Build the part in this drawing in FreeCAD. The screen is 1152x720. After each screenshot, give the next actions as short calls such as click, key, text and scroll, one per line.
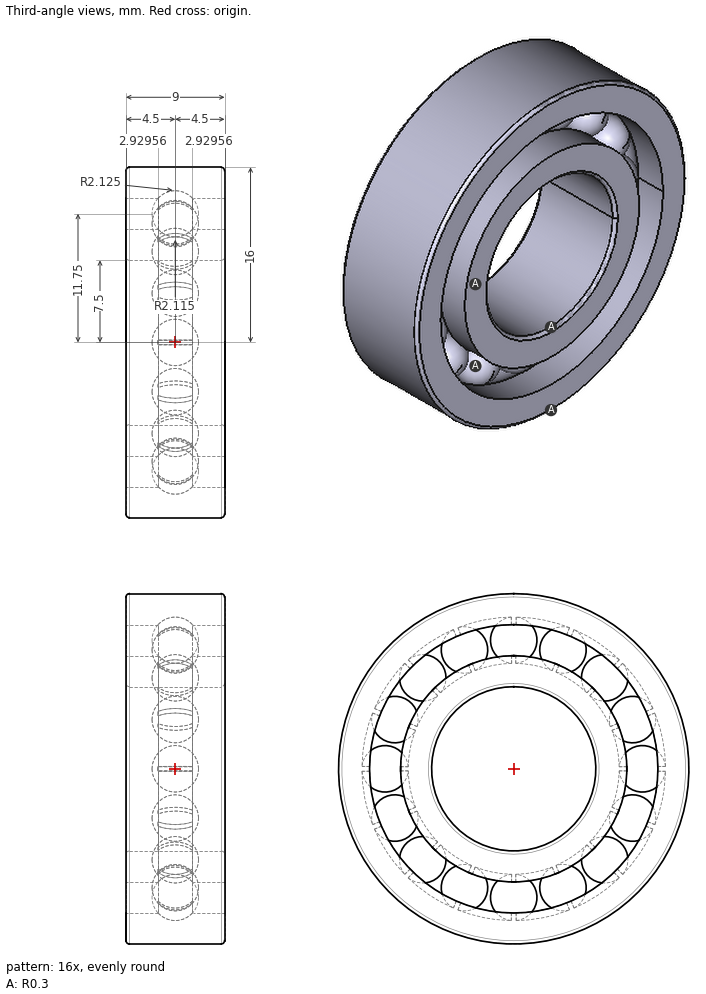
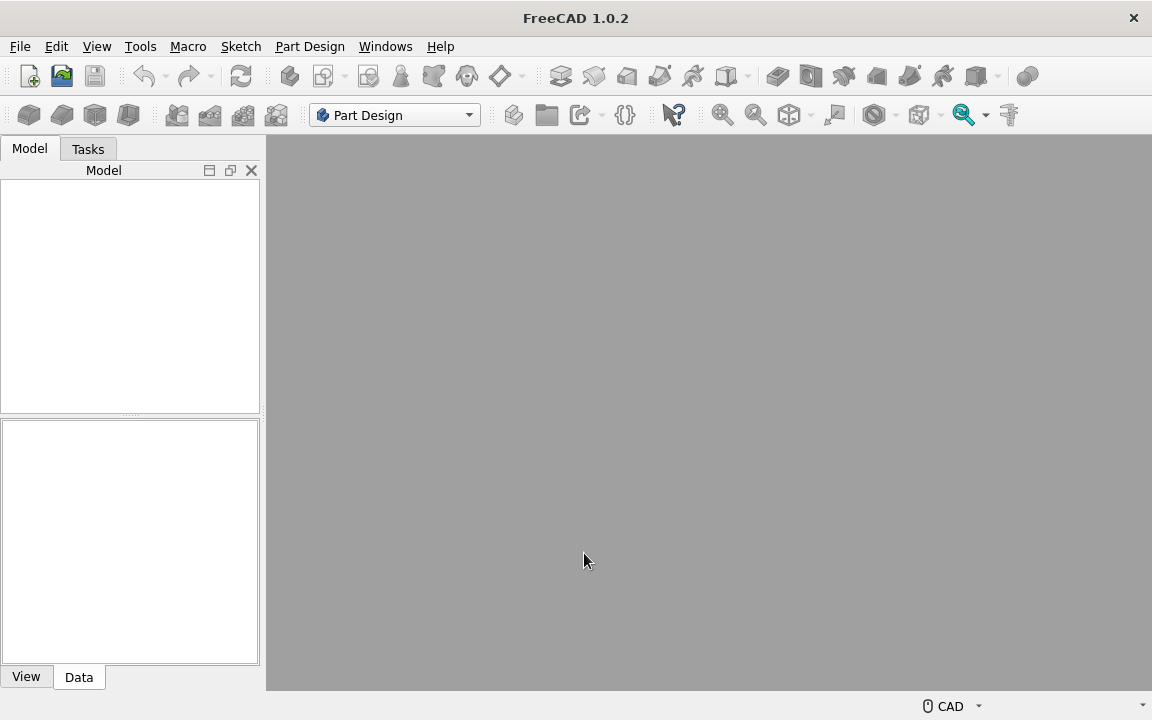
click(29, 76)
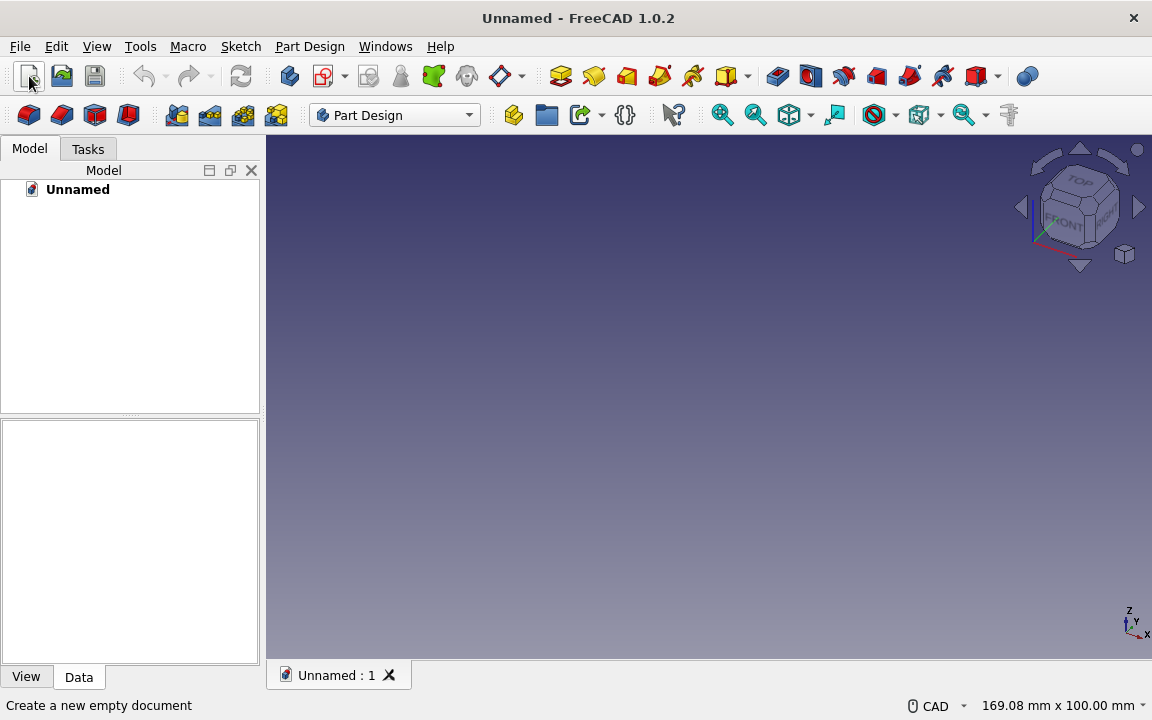
click(322, 76)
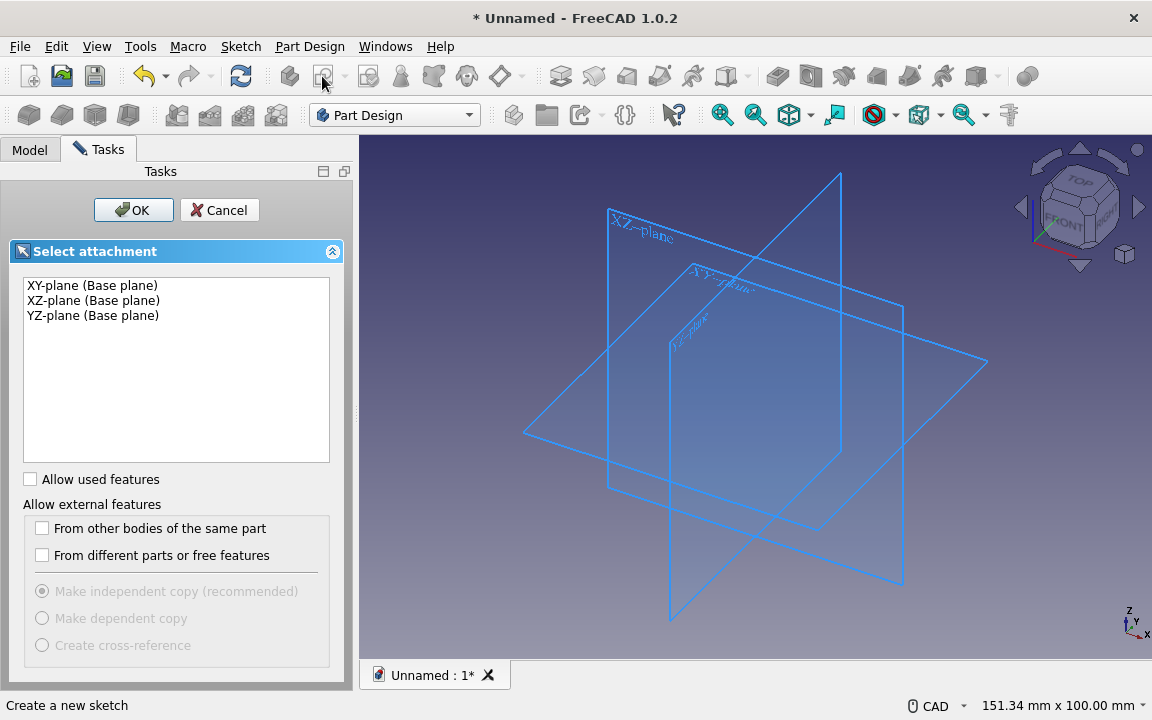
click(84, 286)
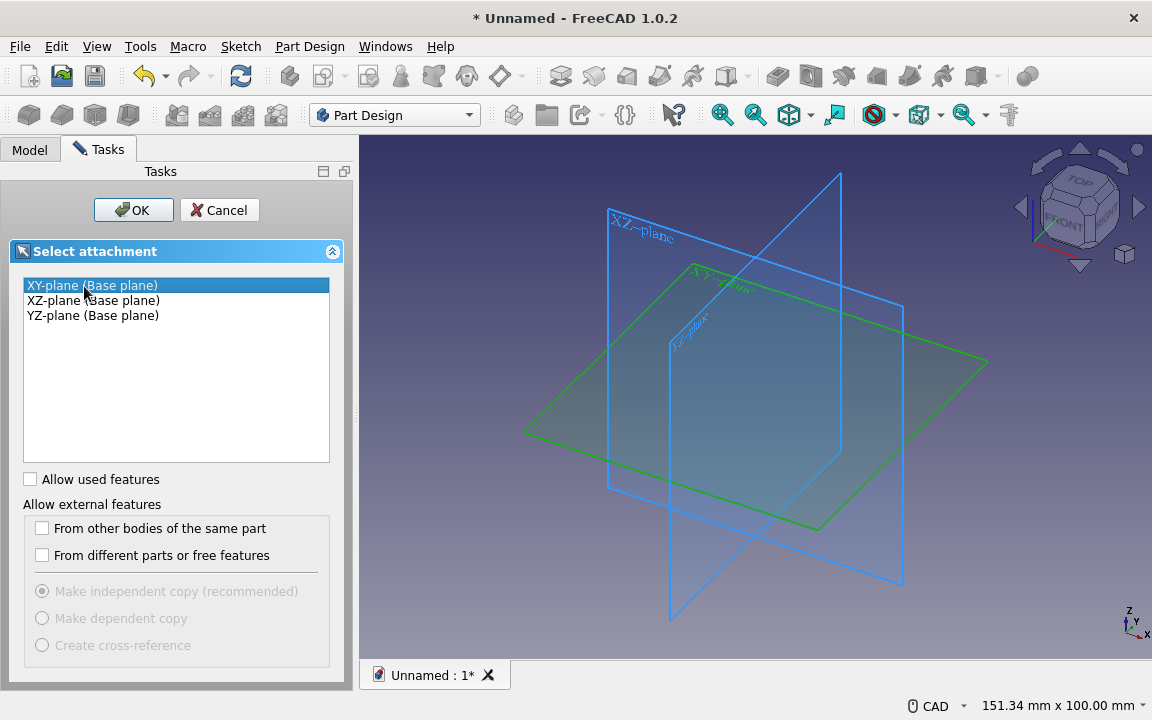
click(134, 210)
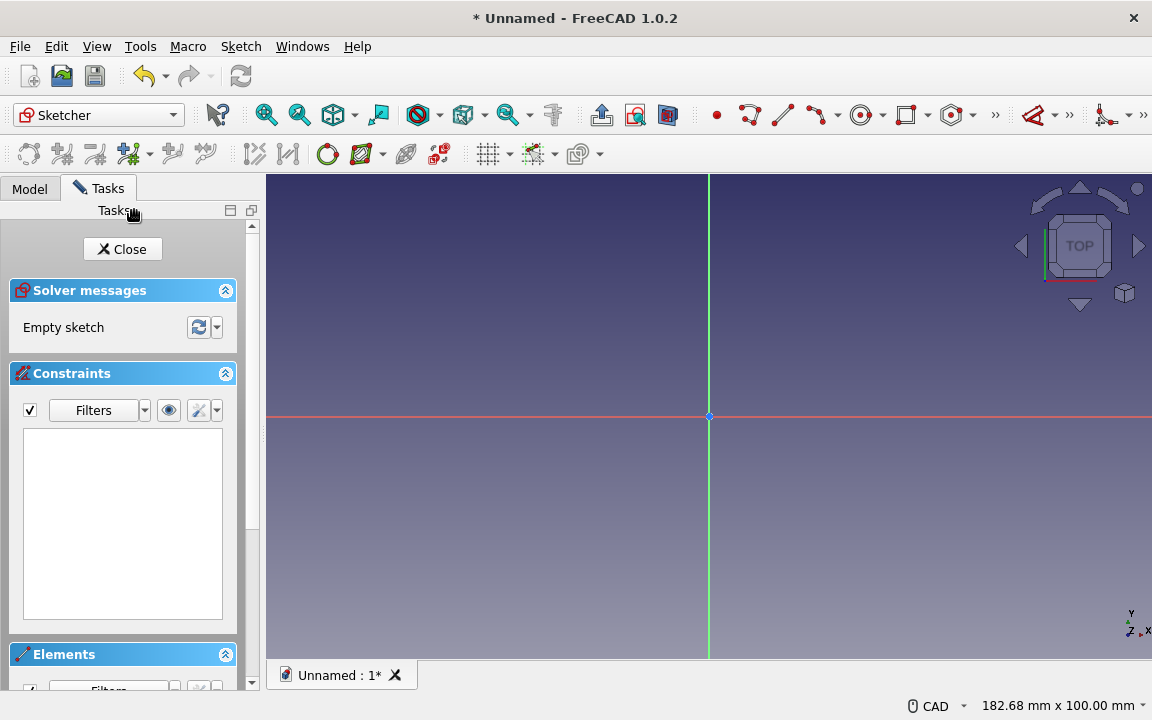
scroll(731, 374, up, 8)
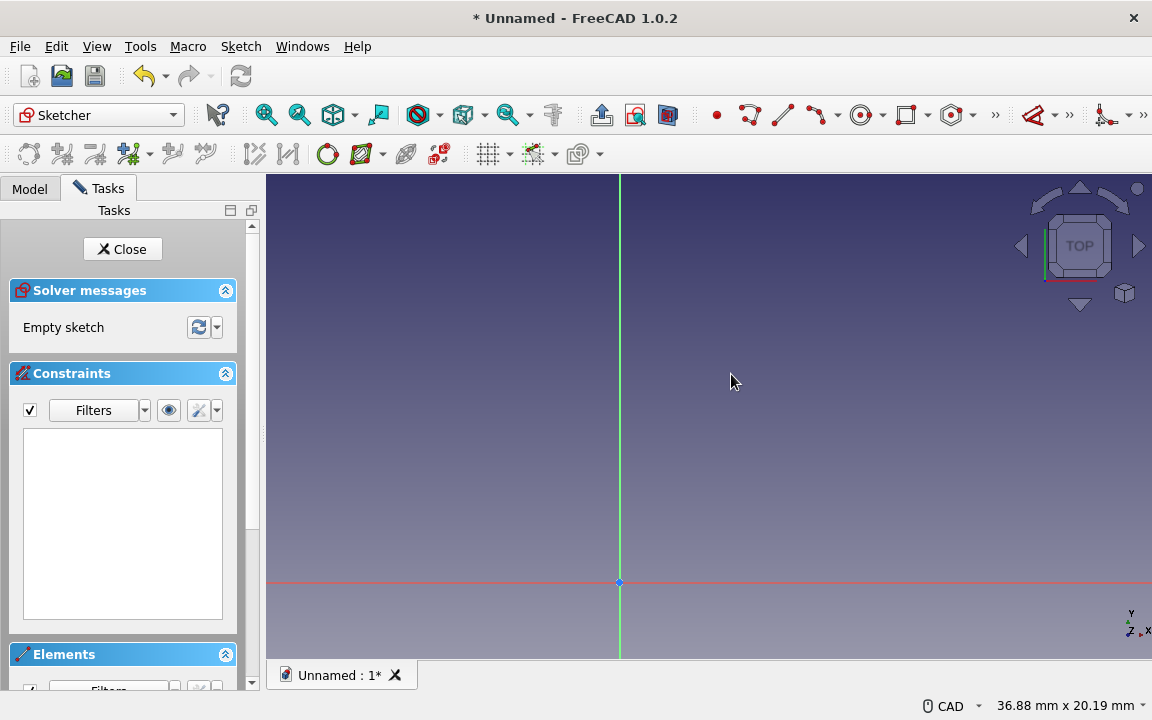
key(g)
key(l)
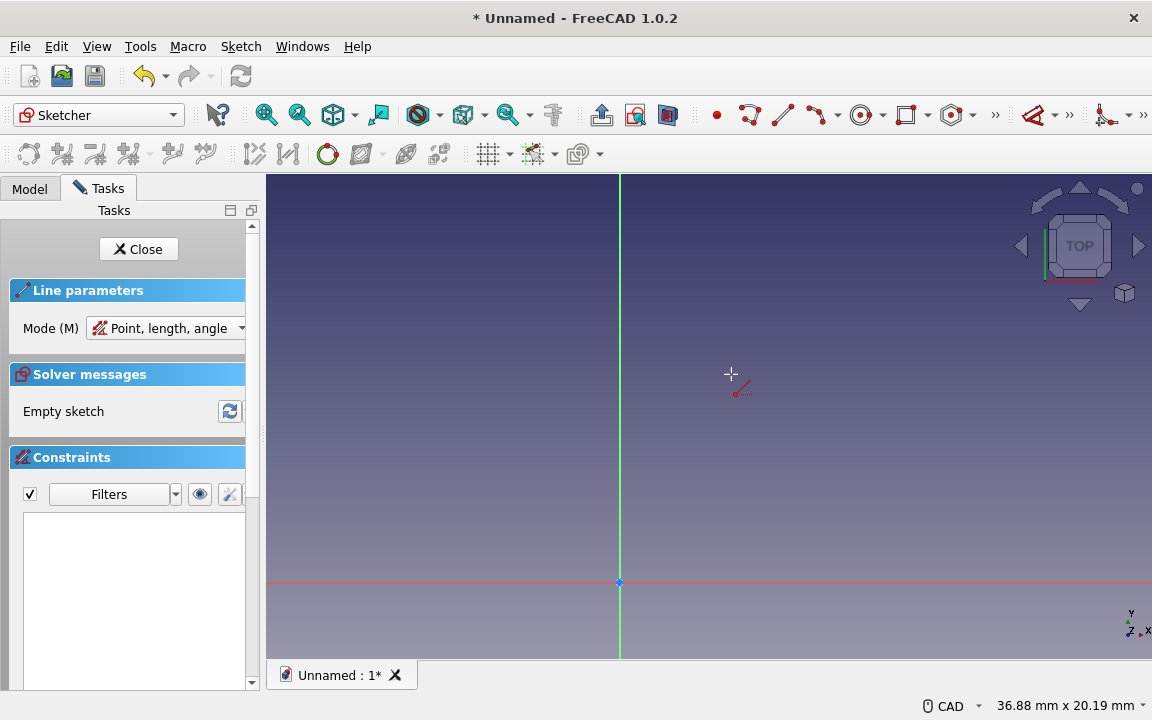
click(569, 301)
click(671, 301)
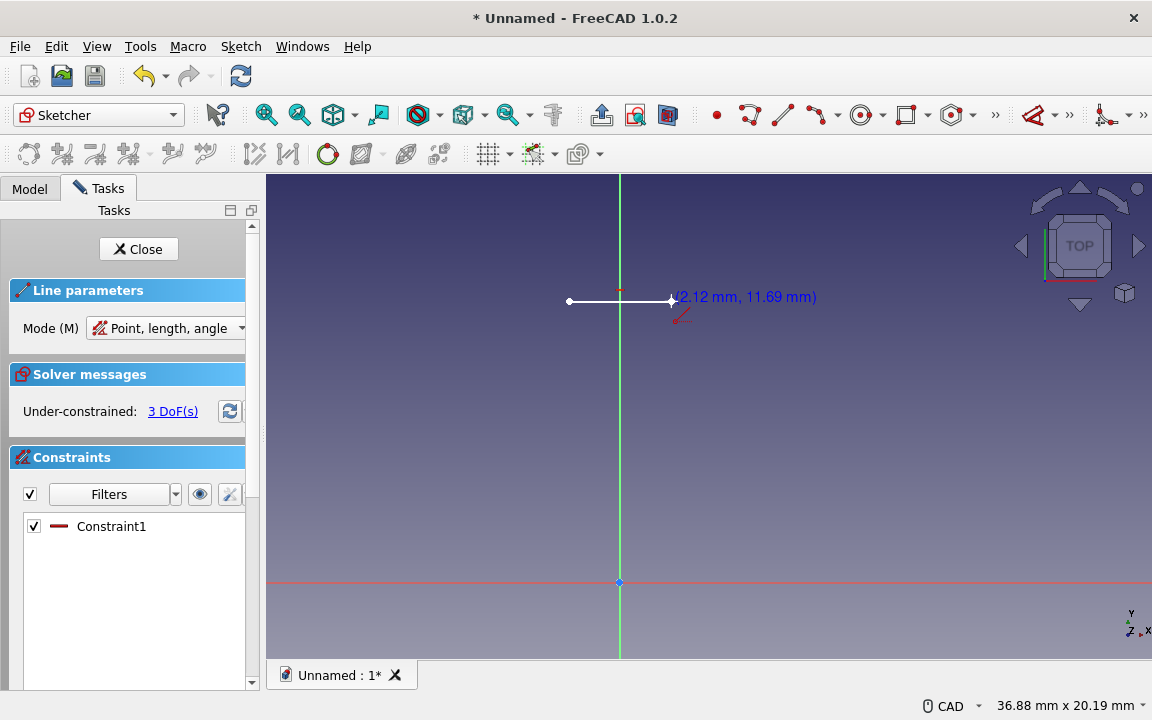
click(816, 116)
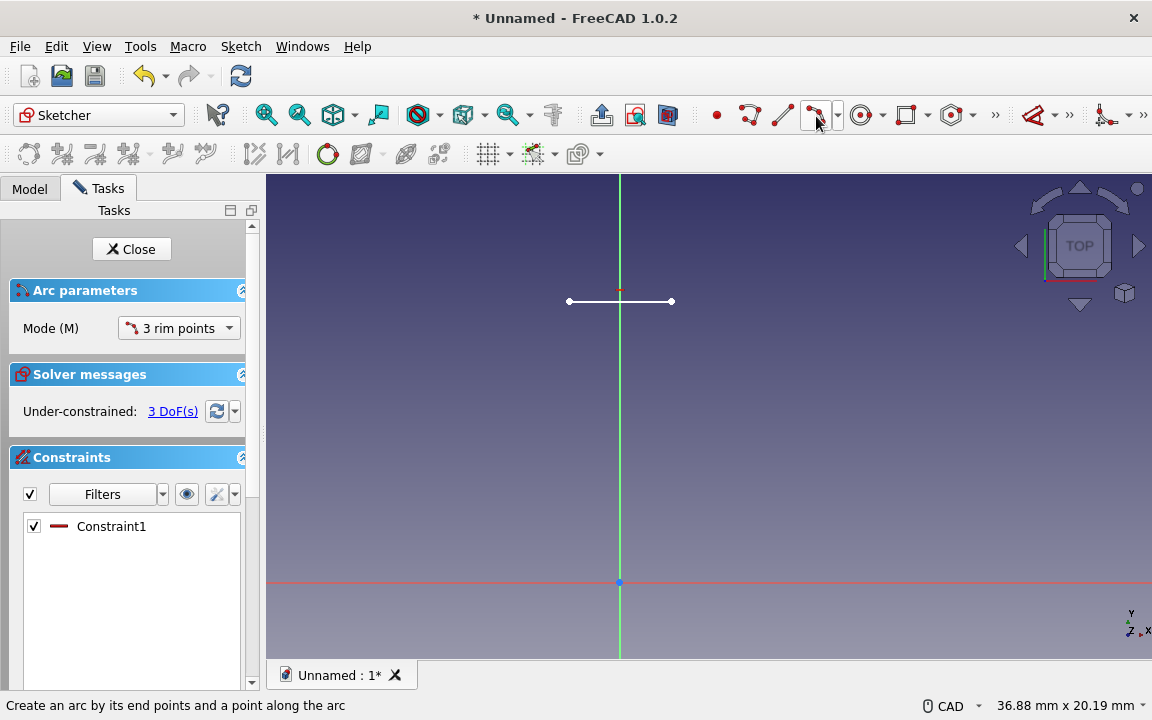
click(671, 302)
click(569, 302)
click(636, 252)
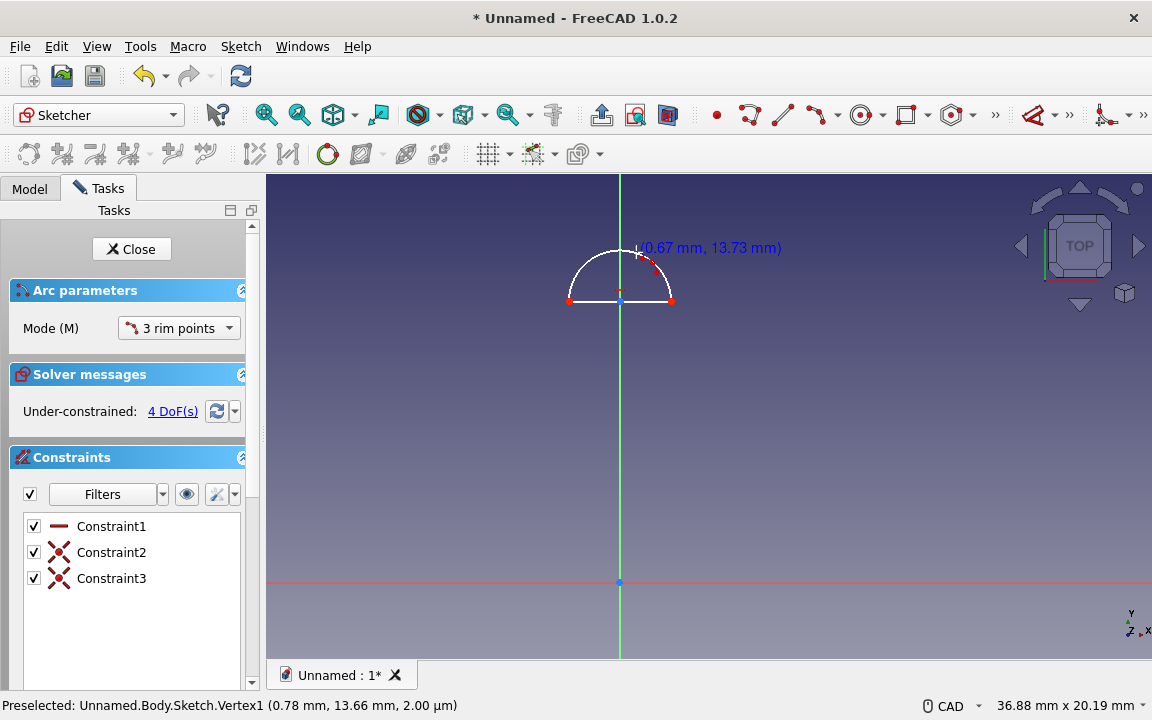
click(783, 116)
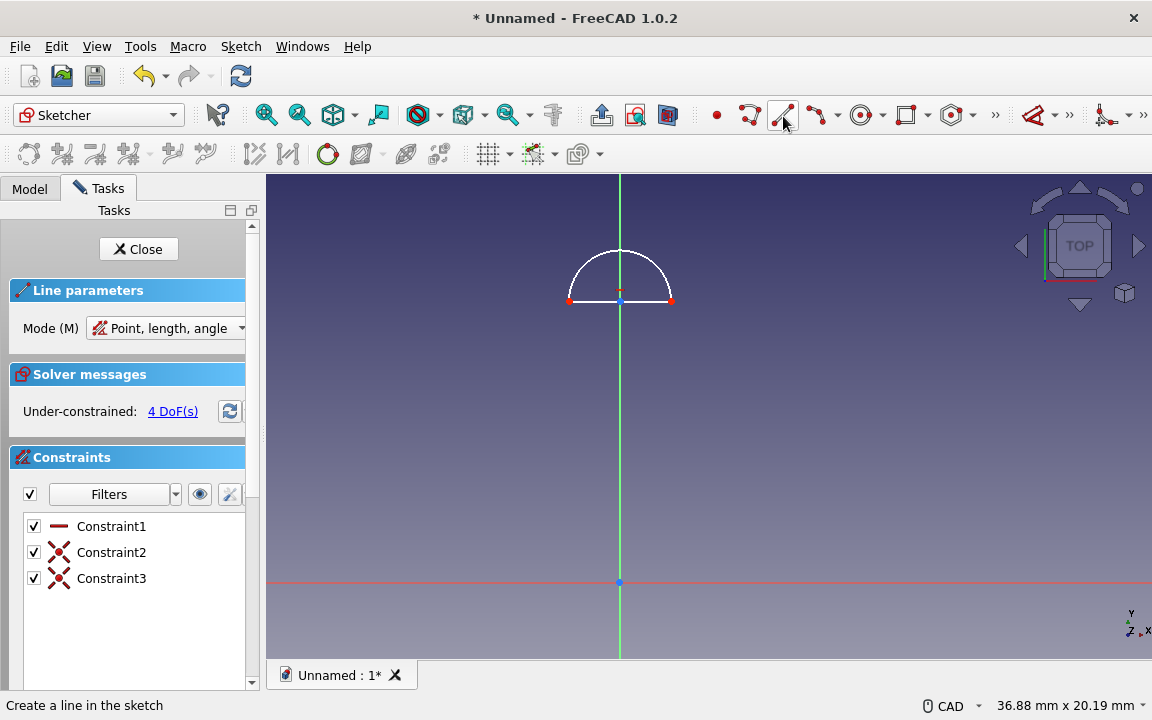
scroll(681, 301, up, 3)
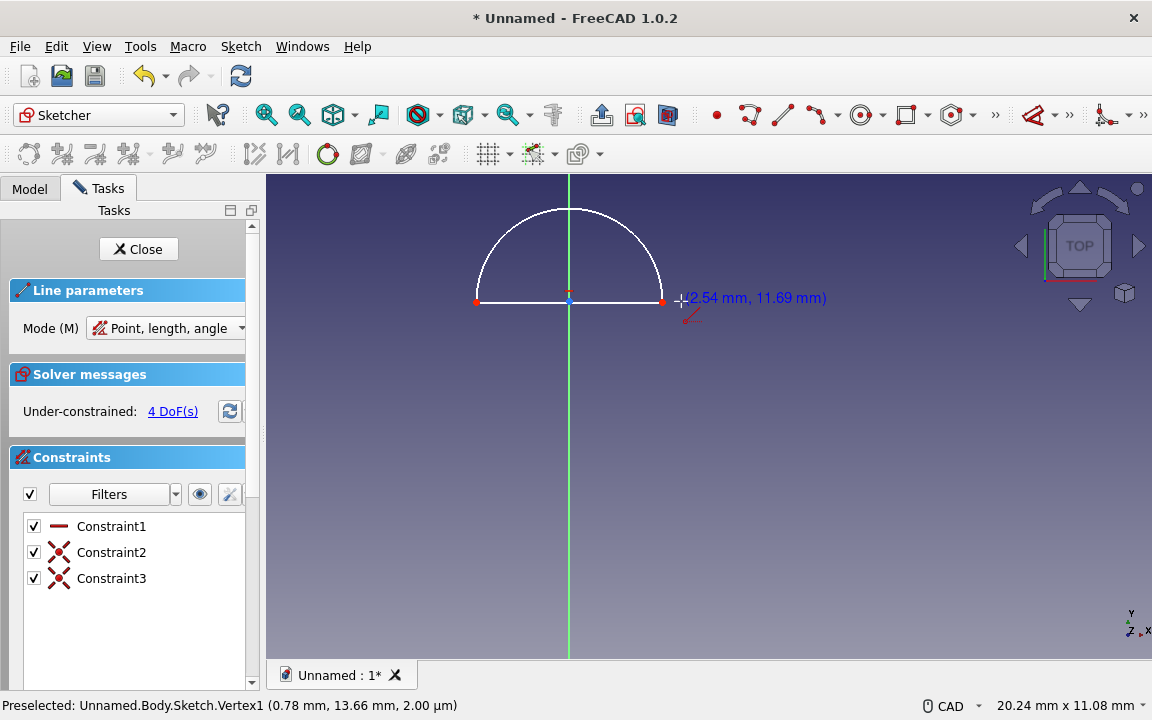
click(681, 300)
click(737, 300)
key(Escape)